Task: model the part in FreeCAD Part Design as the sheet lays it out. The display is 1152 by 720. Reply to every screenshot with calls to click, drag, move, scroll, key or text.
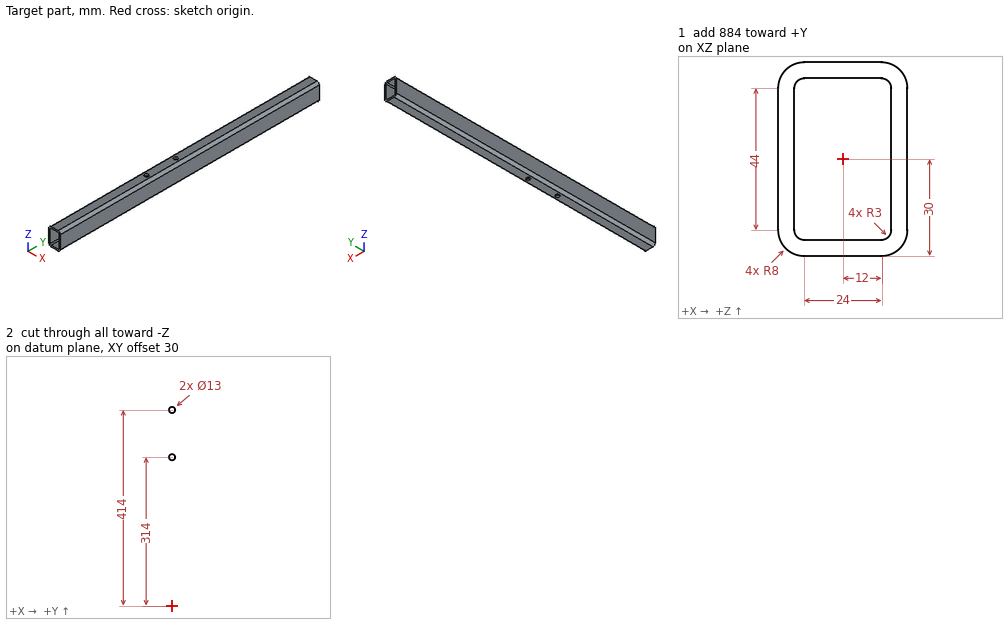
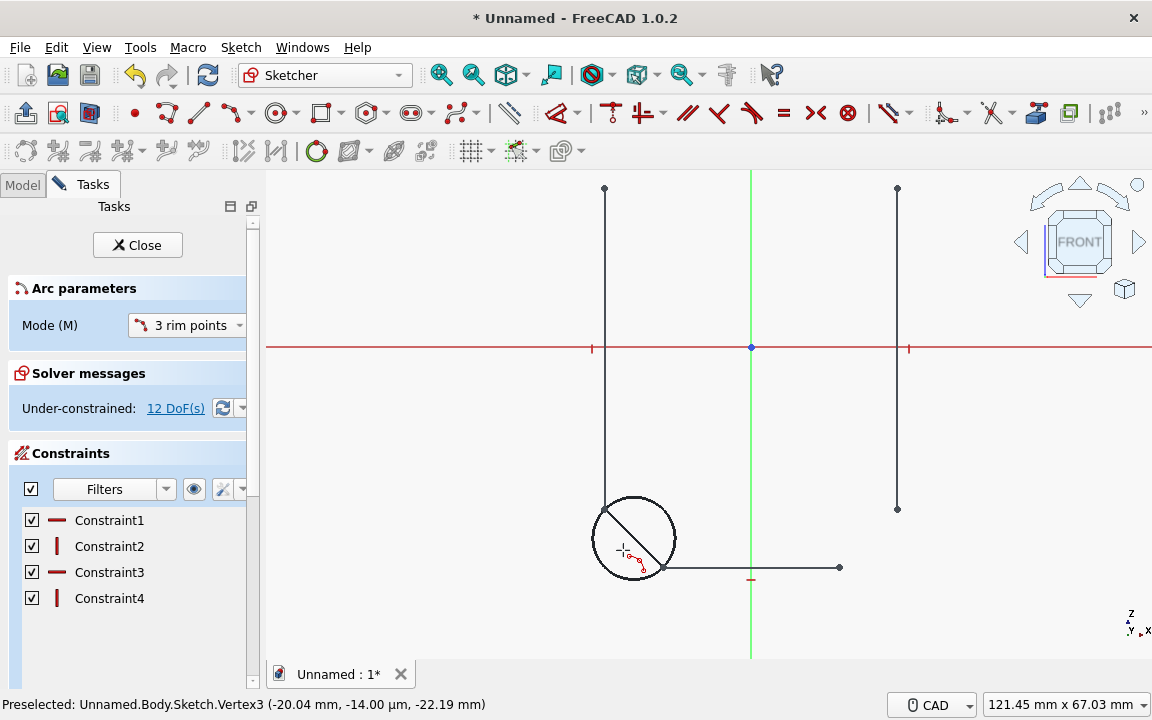
click(622, 549)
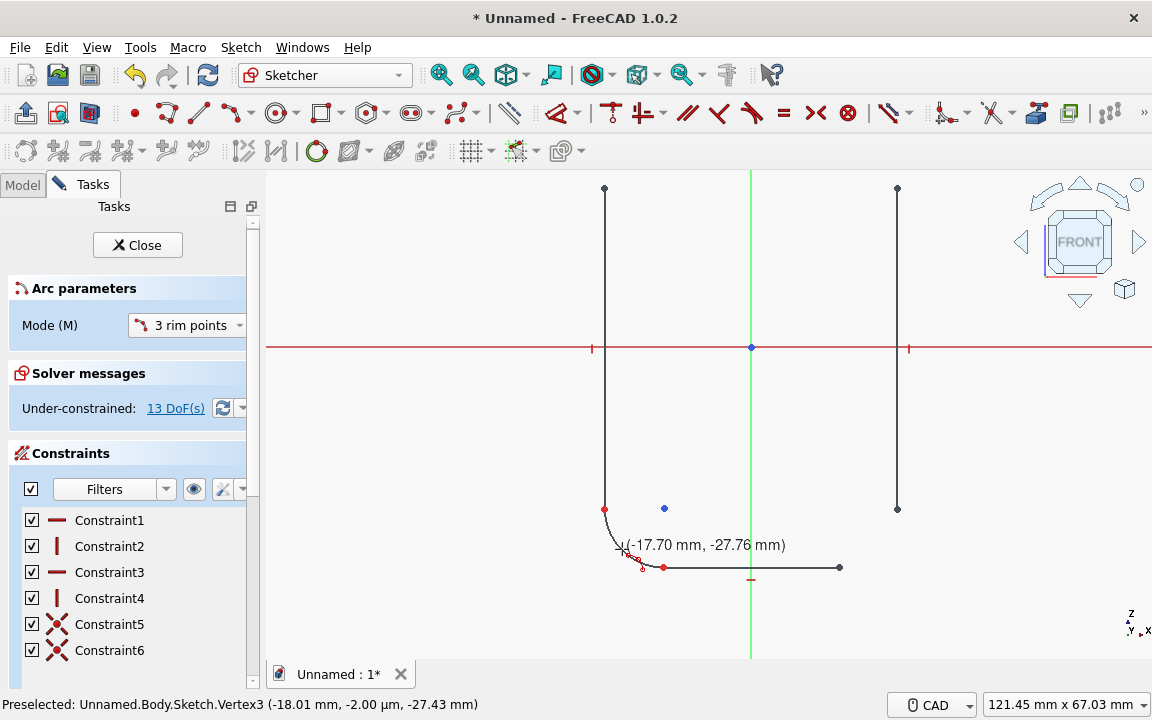
scroll(416, 551, down, 2)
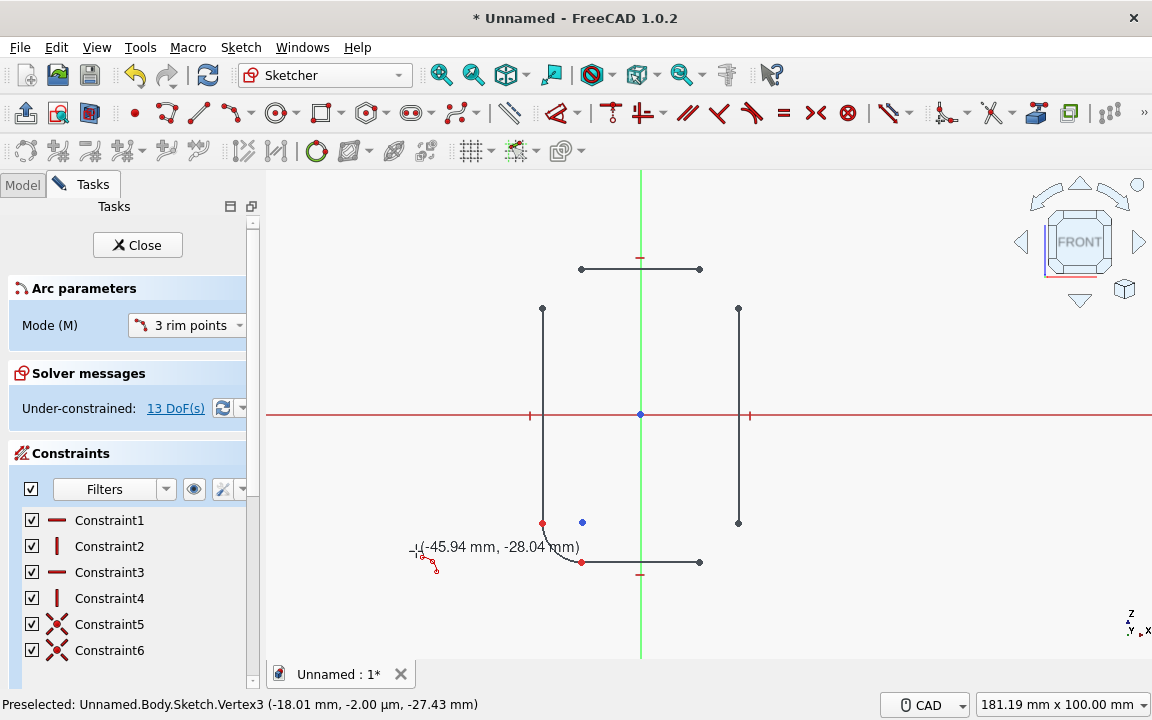
click(543, 308)
click(582, 269)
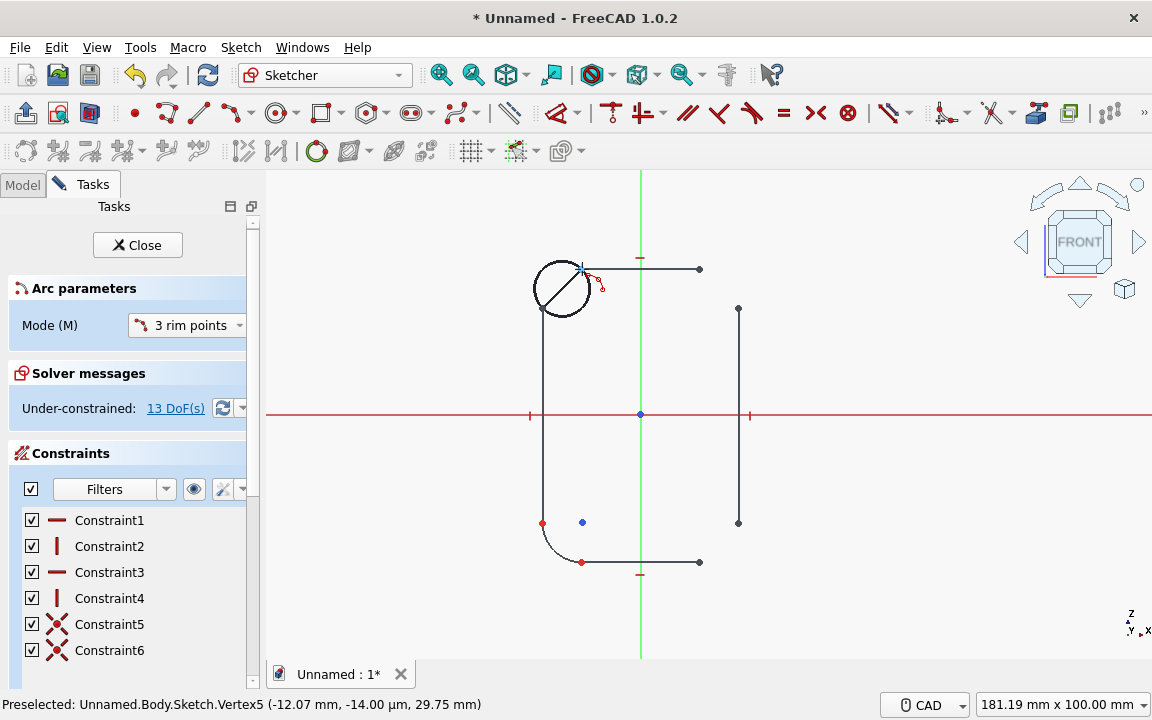
scroll(554, 280, up, 2)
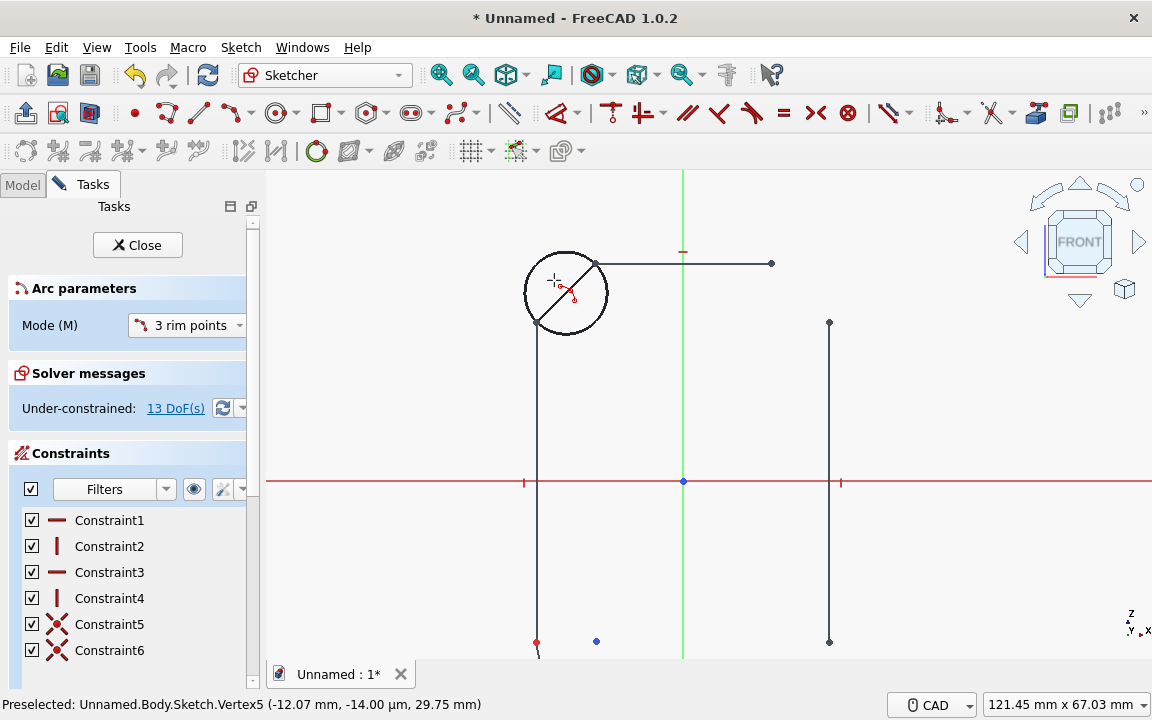
click(554, 279)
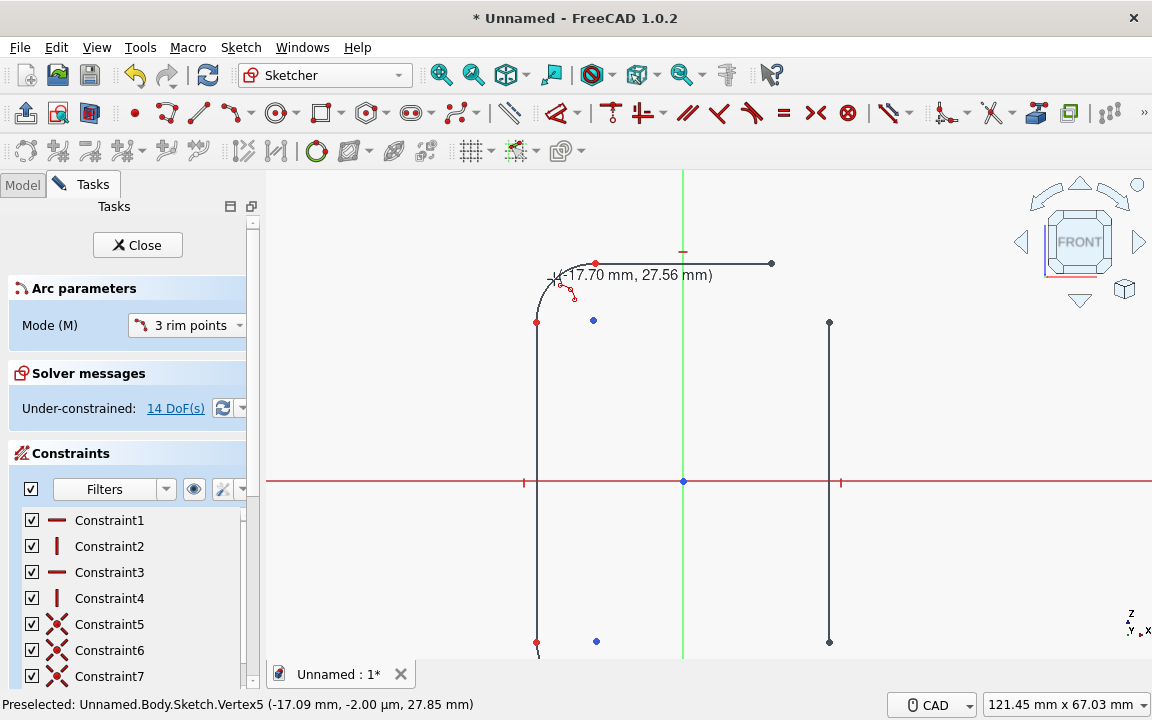
click(771, 264)
click(829, 322)
click(812, 279)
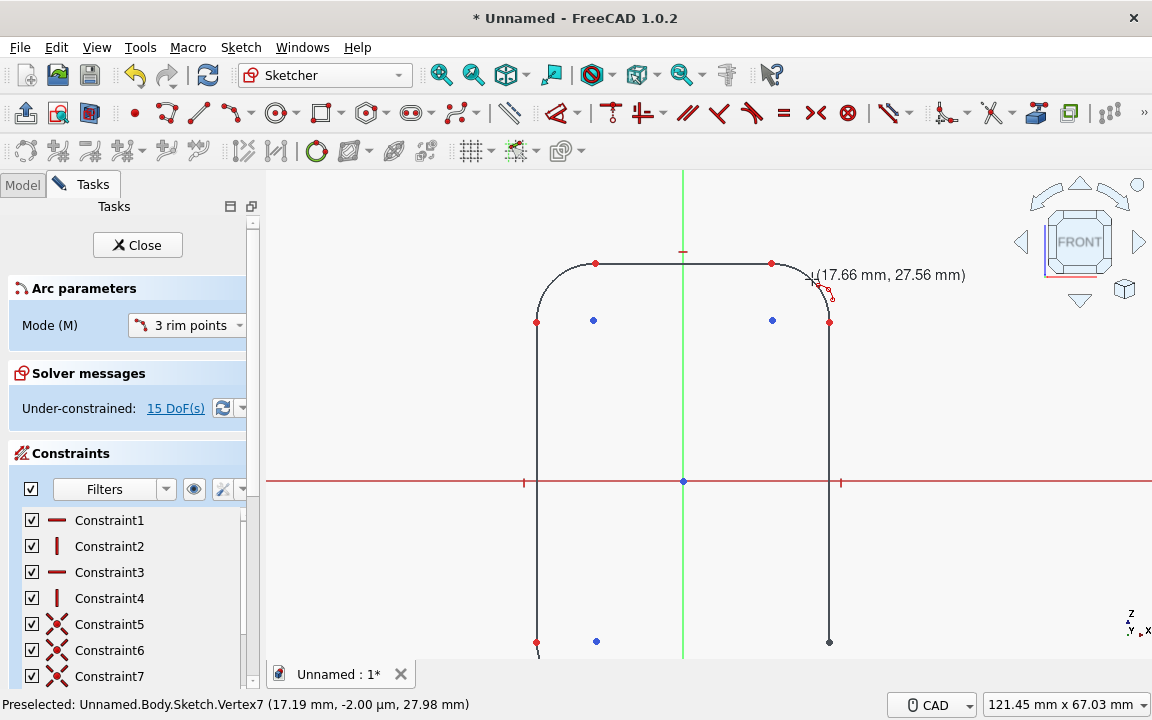
scroll(554, 279, down, 2)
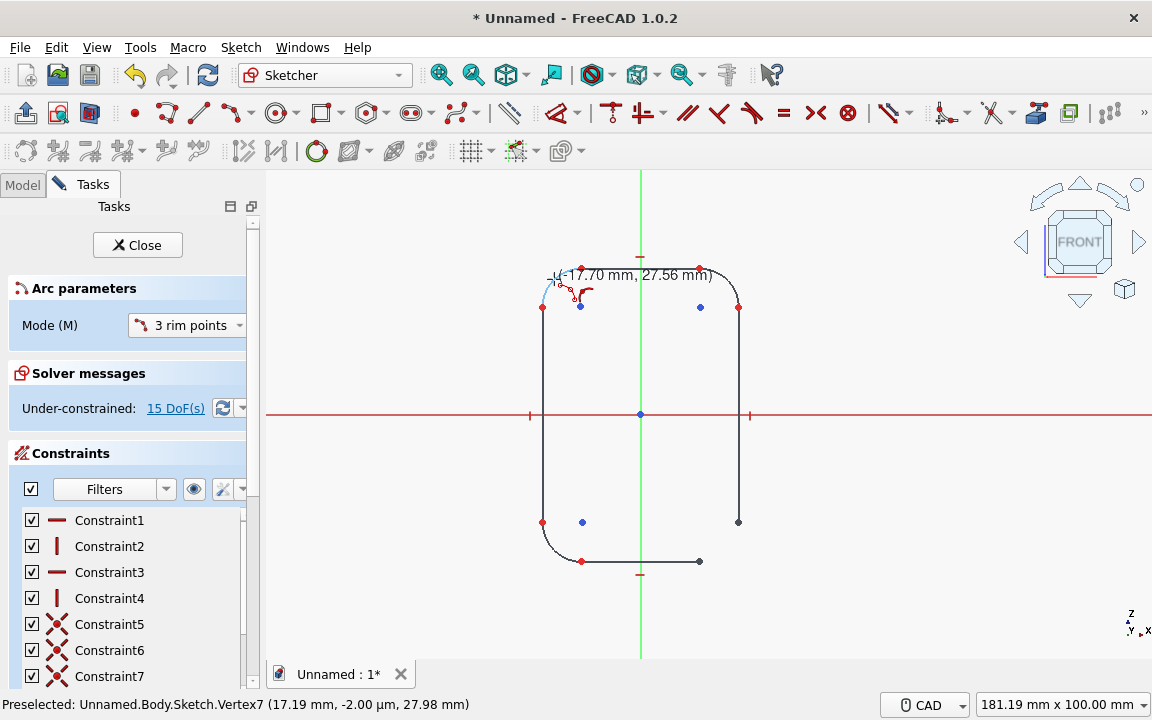
click(739, 523)
click(700, 562)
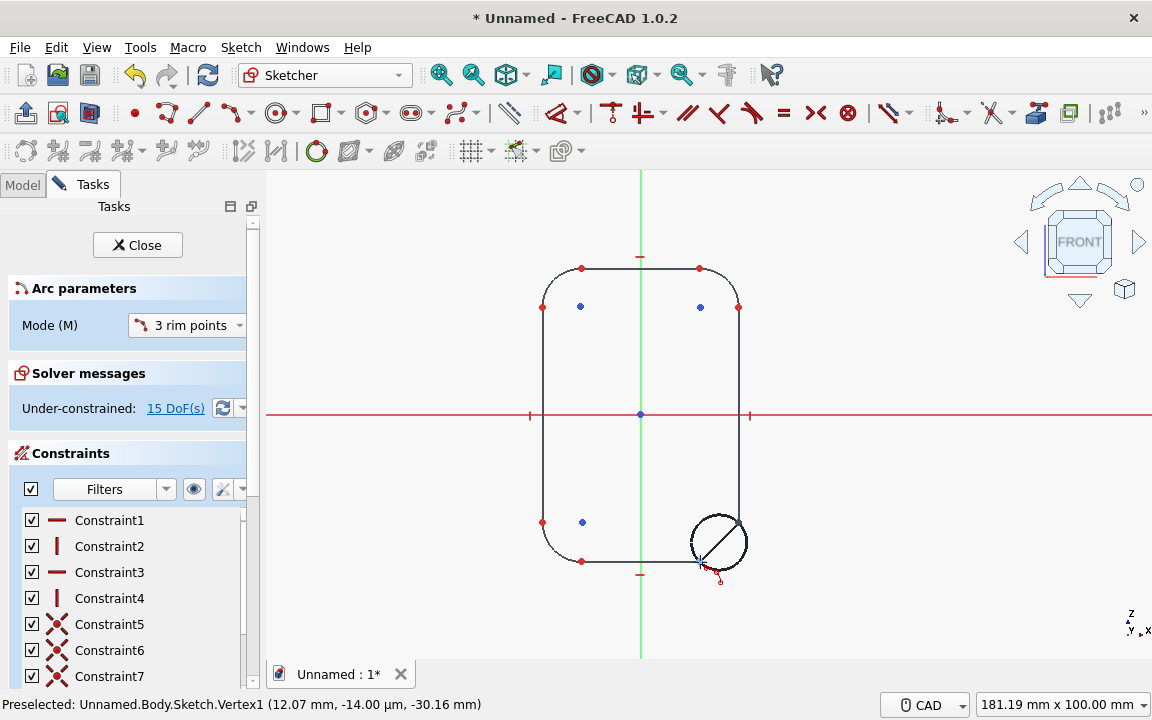
scroll(727, 550, up, 2)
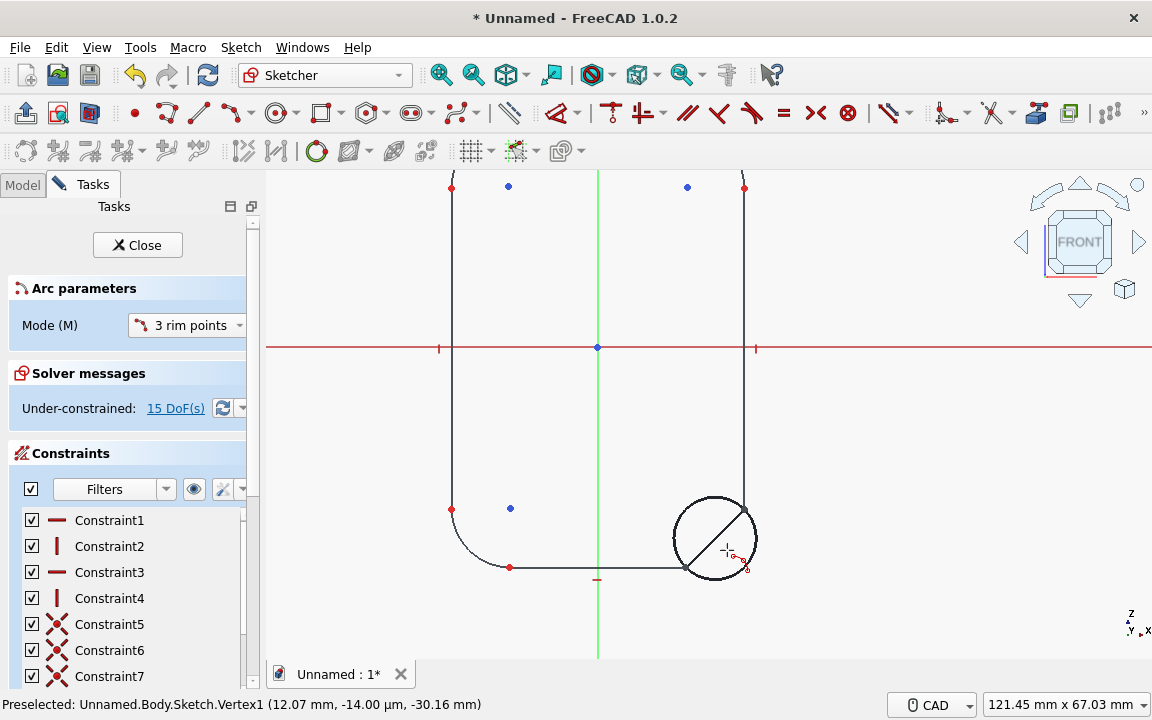
click(727, 549)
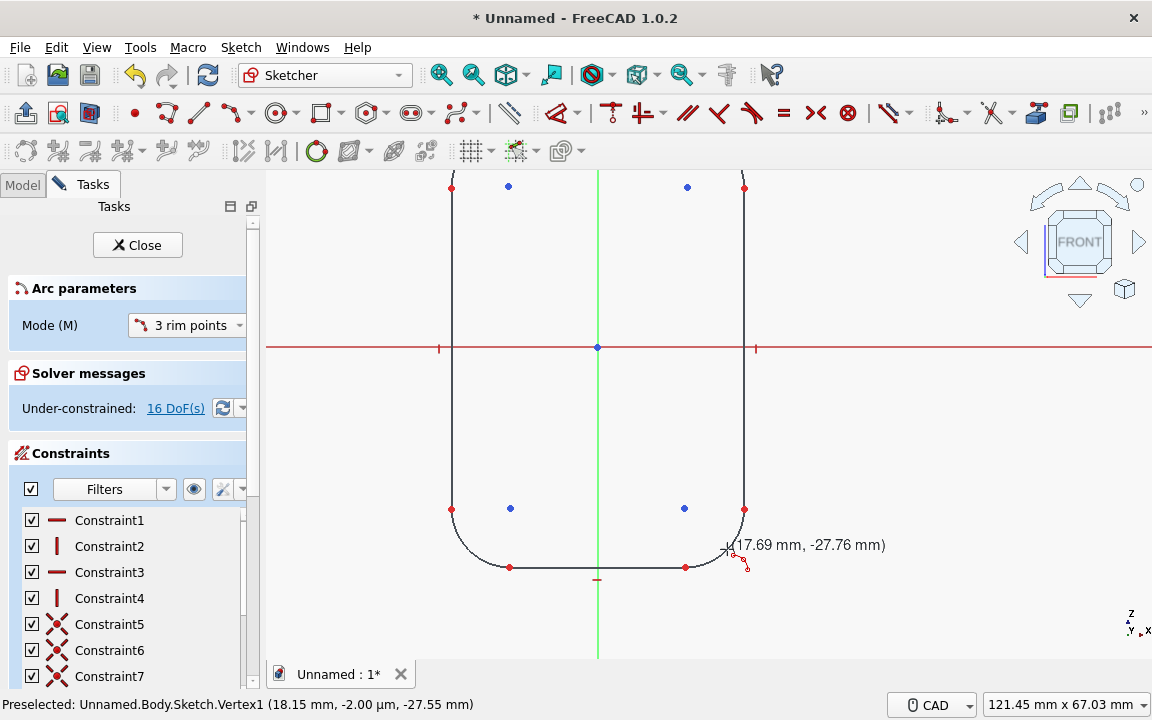
click(200, 114)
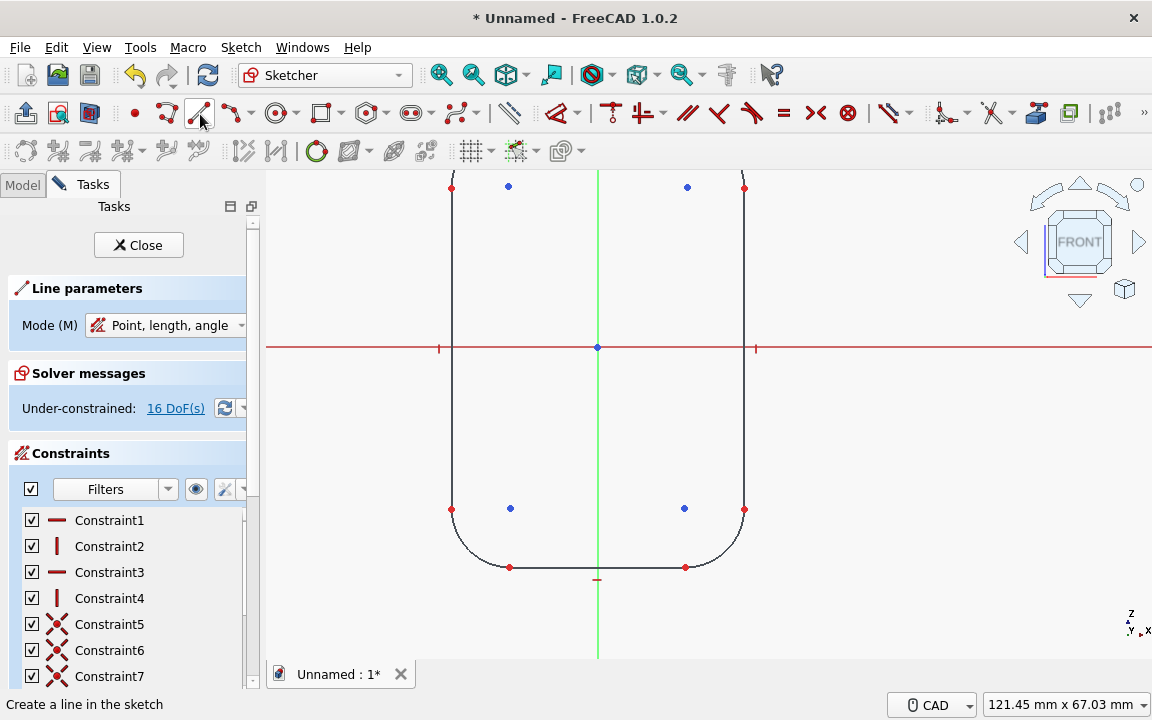
click(510, 530)
click(686, 530)